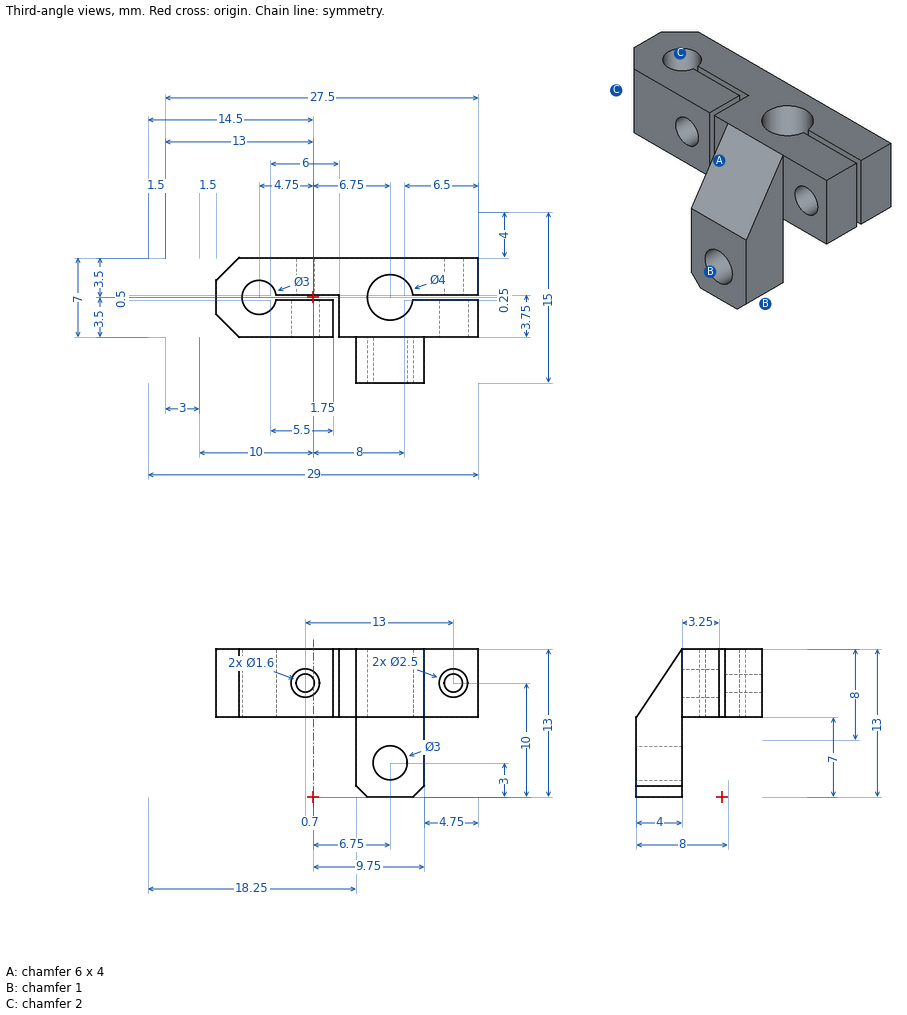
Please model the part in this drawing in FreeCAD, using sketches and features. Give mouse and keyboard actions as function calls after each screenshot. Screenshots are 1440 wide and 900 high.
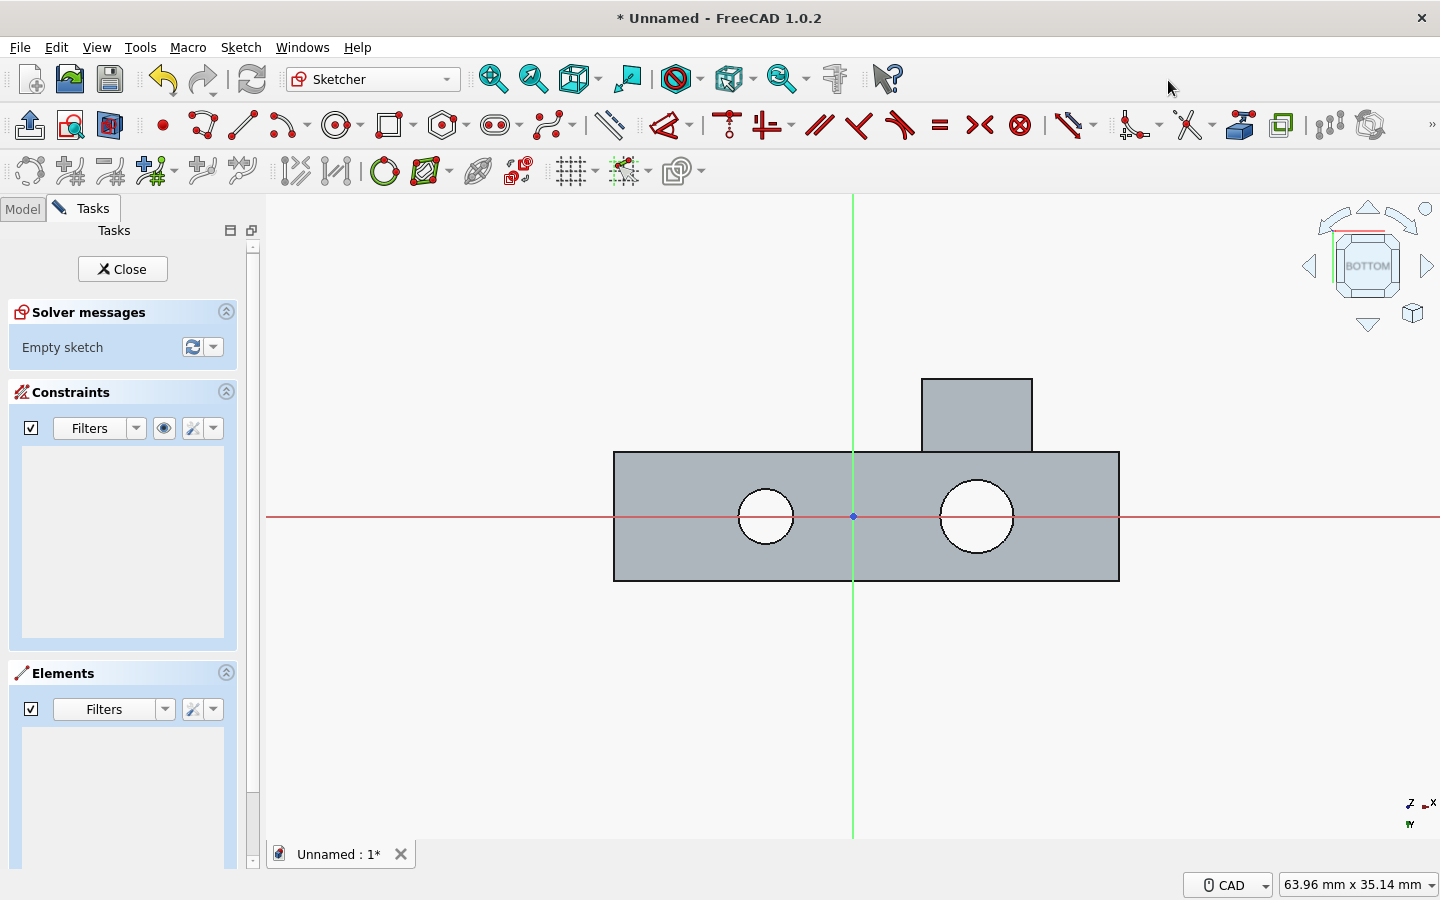
scroll(1088, 462, up, 4)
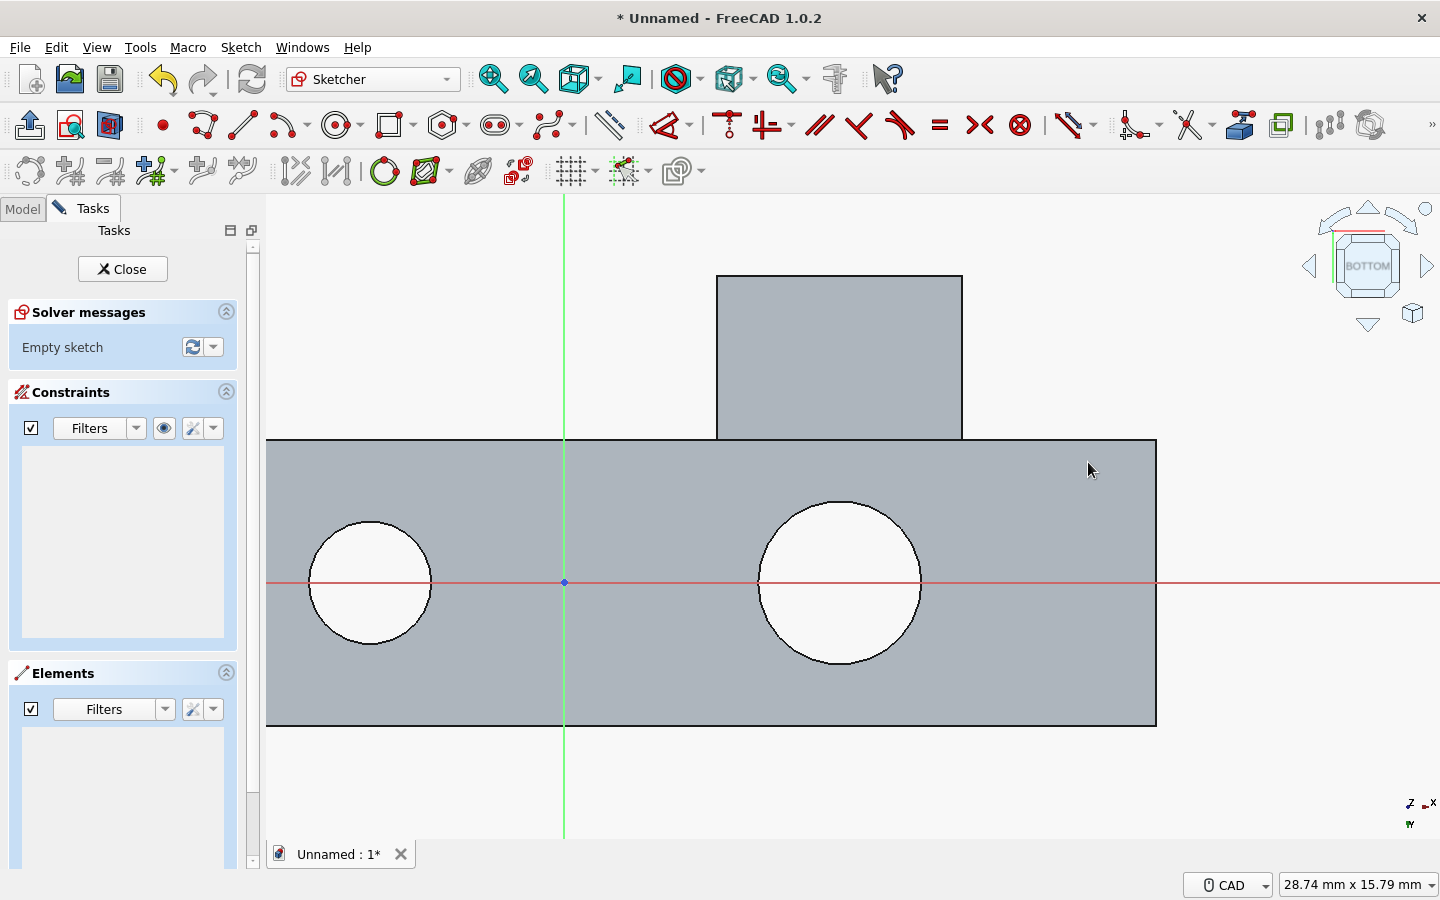
click(204, 126)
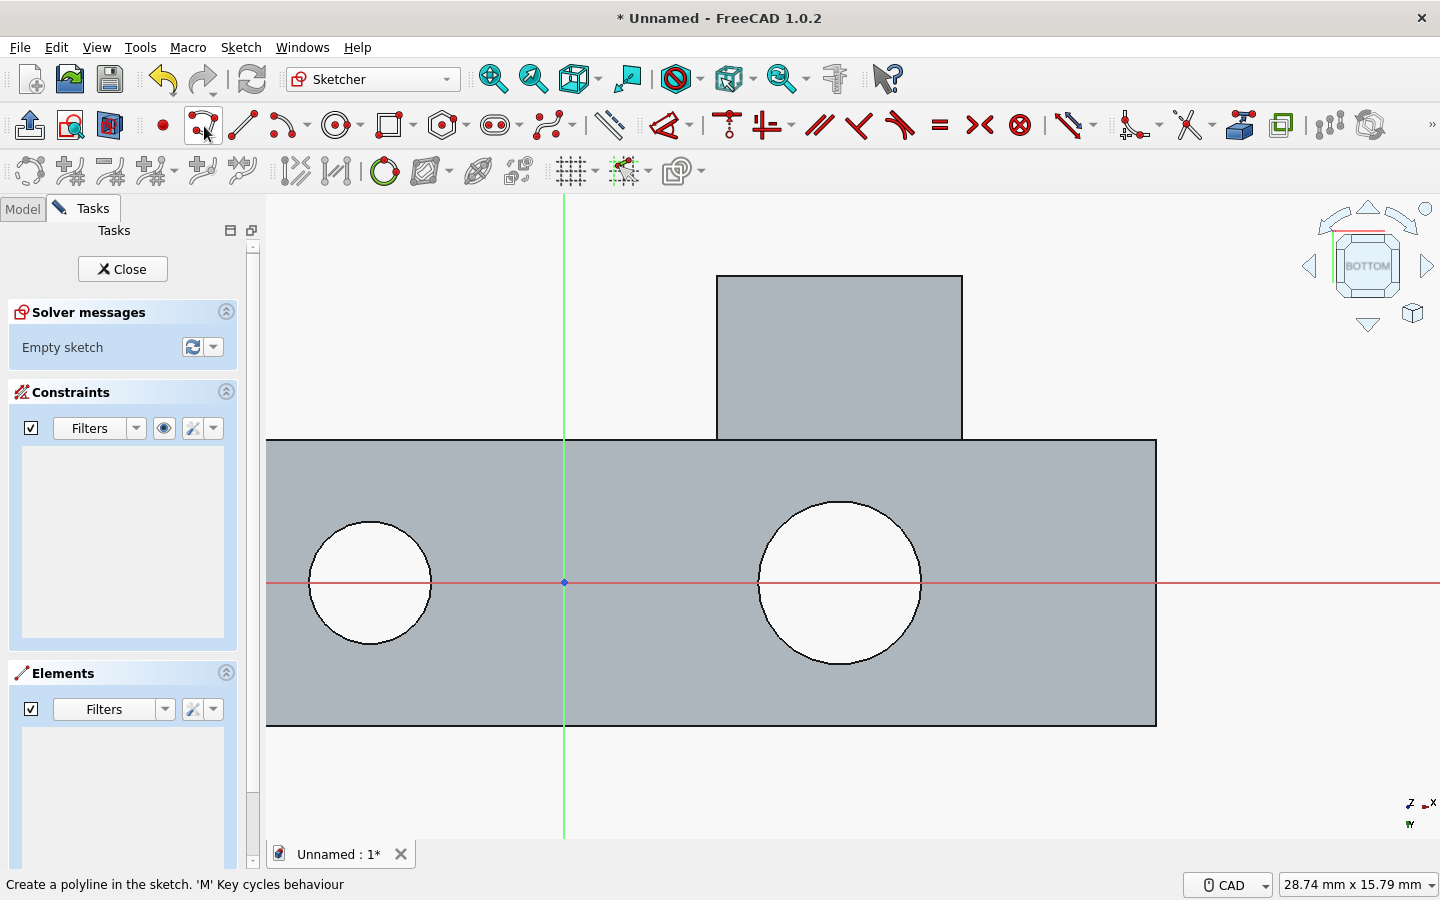
scroll(636, 573, up, 3)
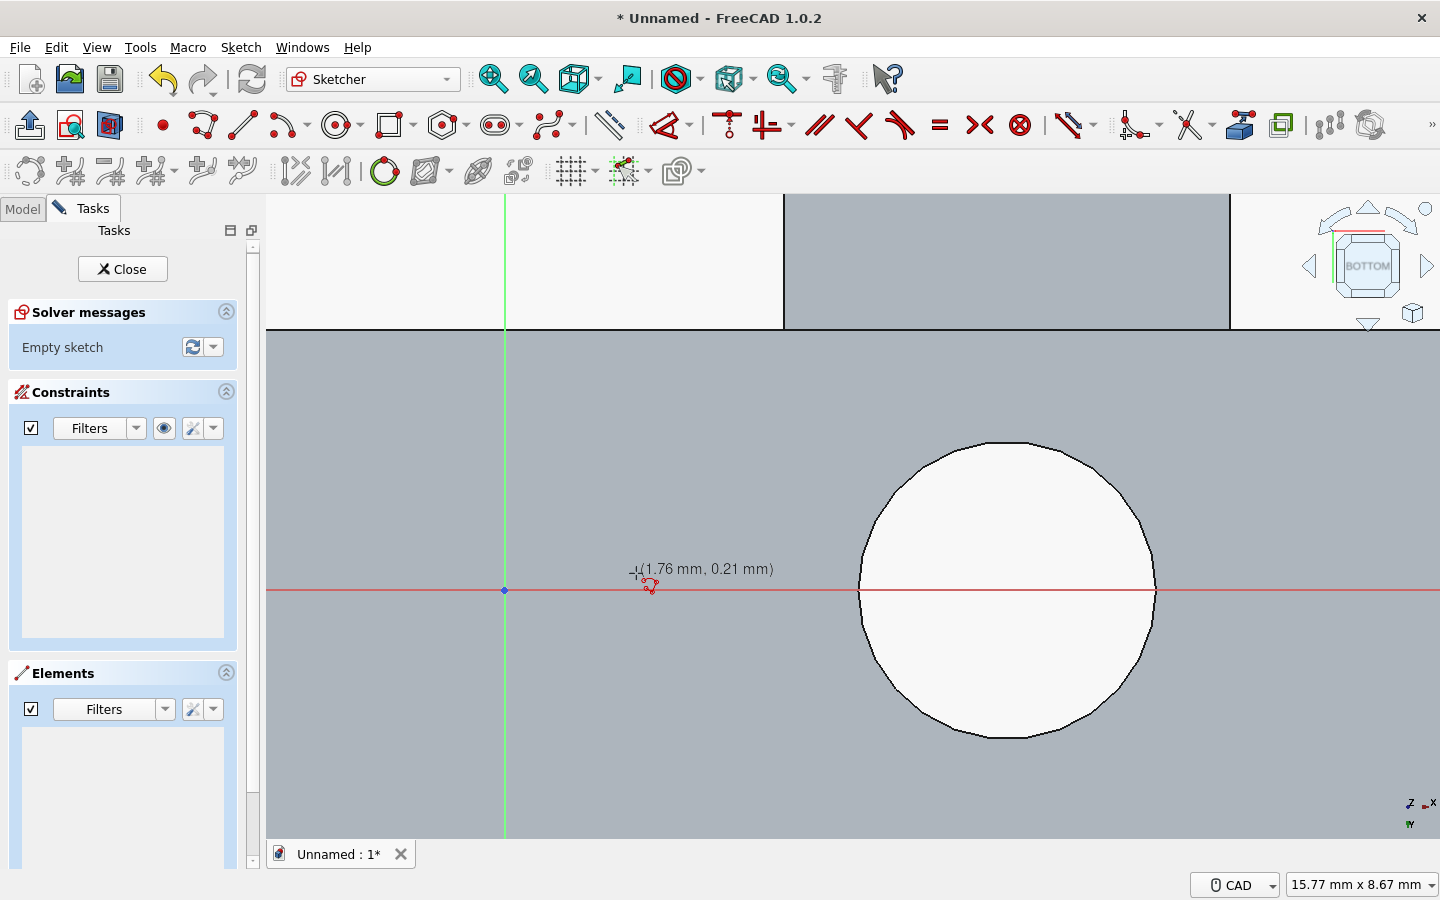
click(635, 572)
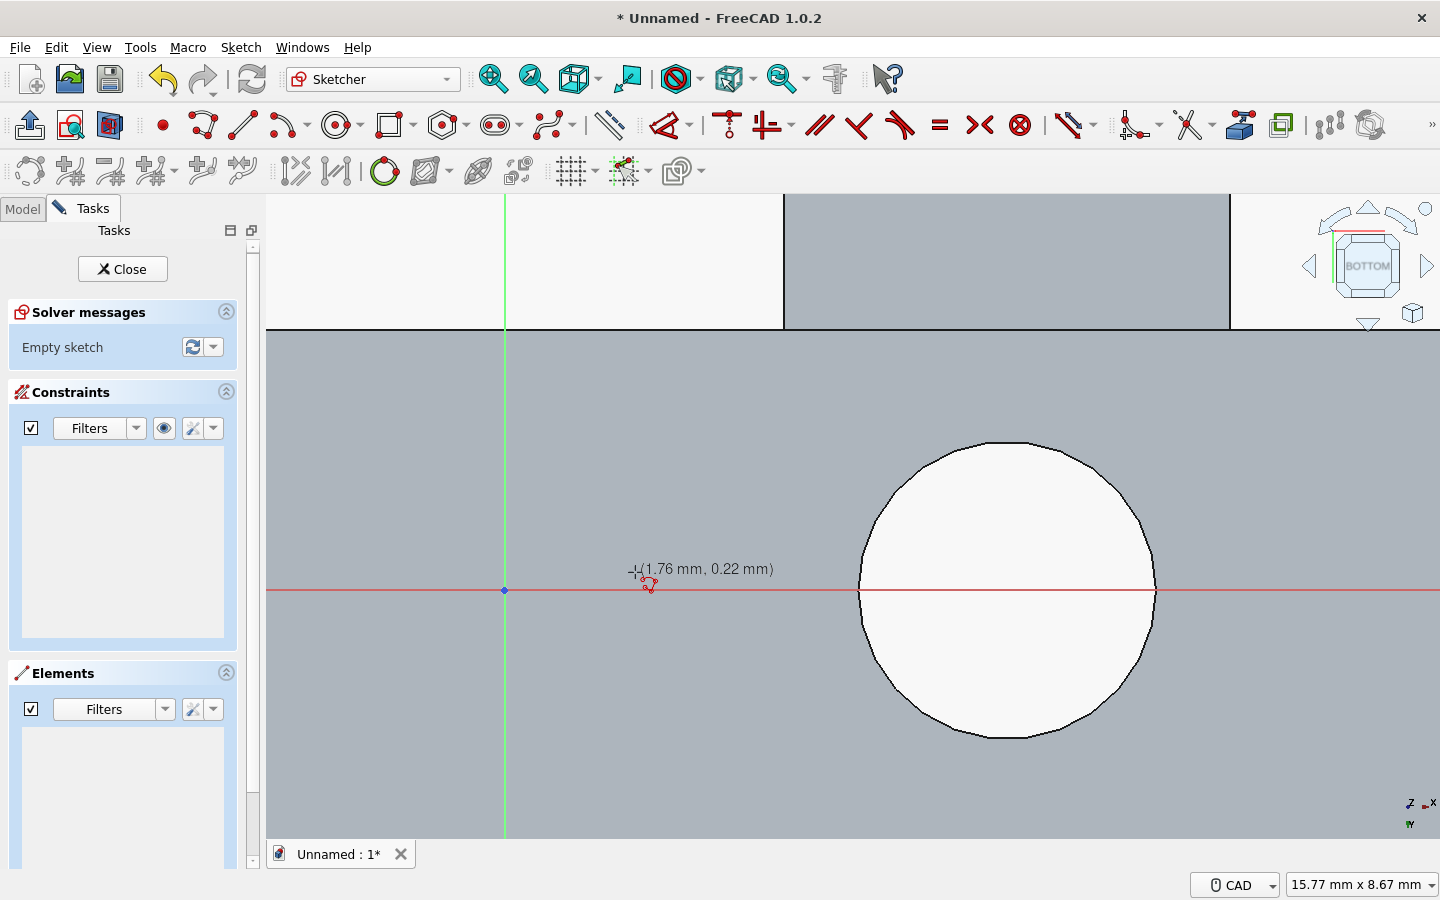
scroll(638, 574, down, 3)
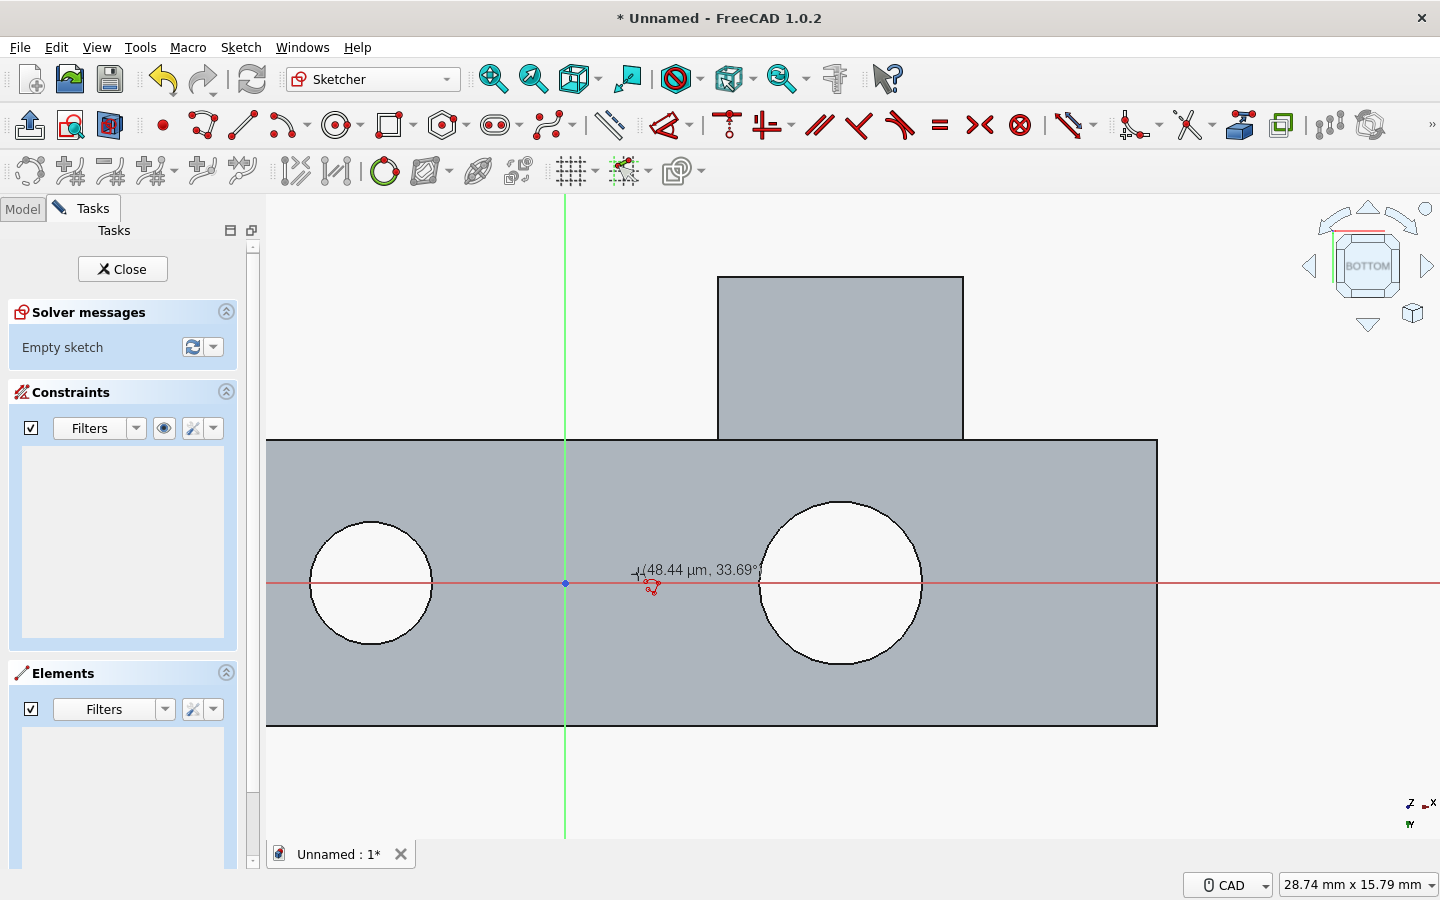
scroll(412, 573, up, 3)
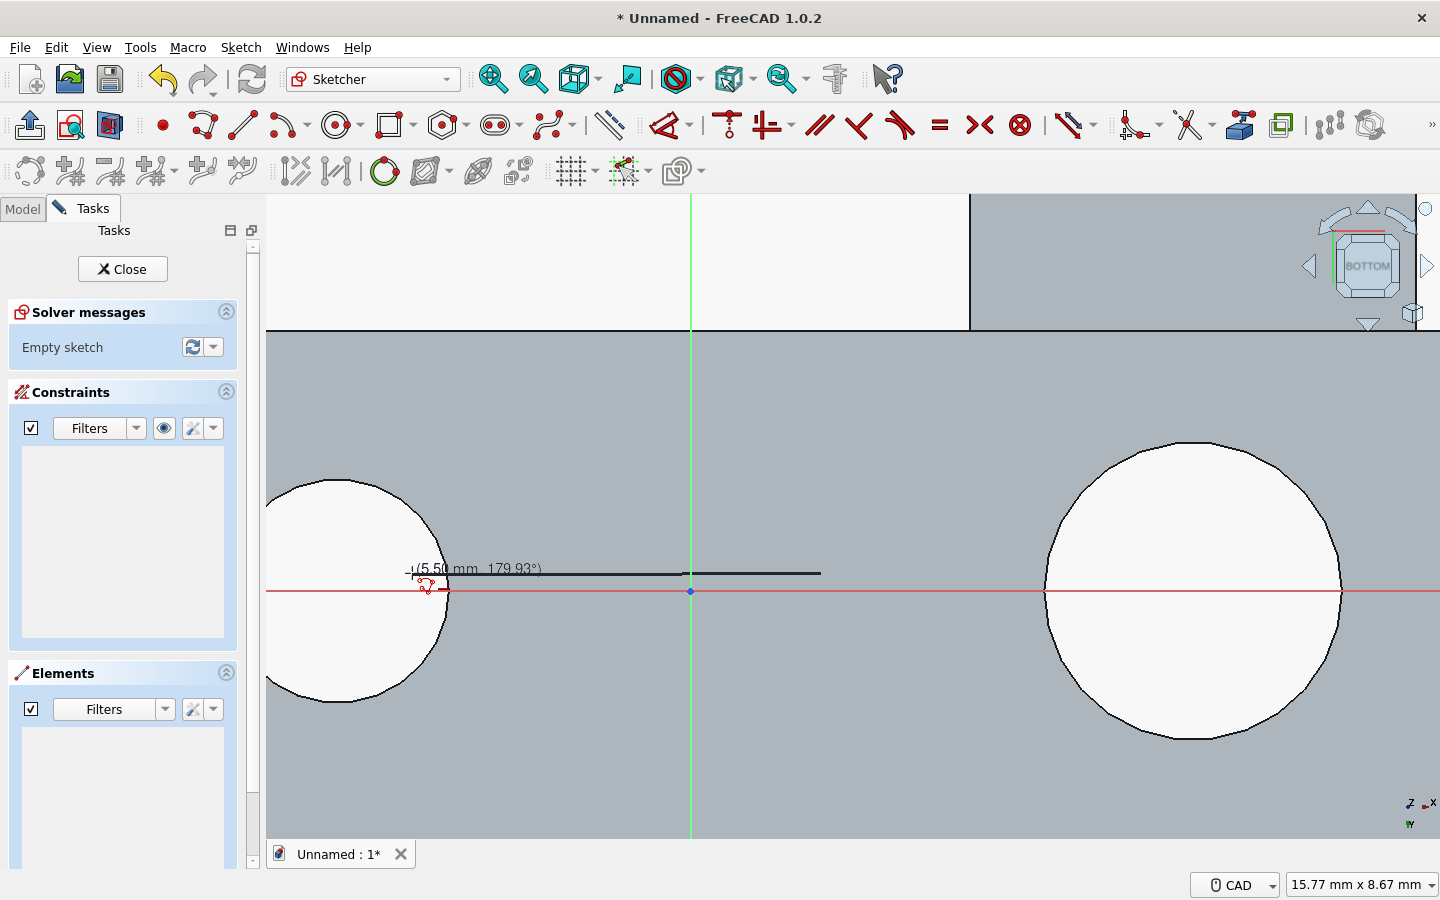
click(412, 573)
click(412, 610)
click(858, 610)
click(858, 331)
click(821, 331)
click(821, 574)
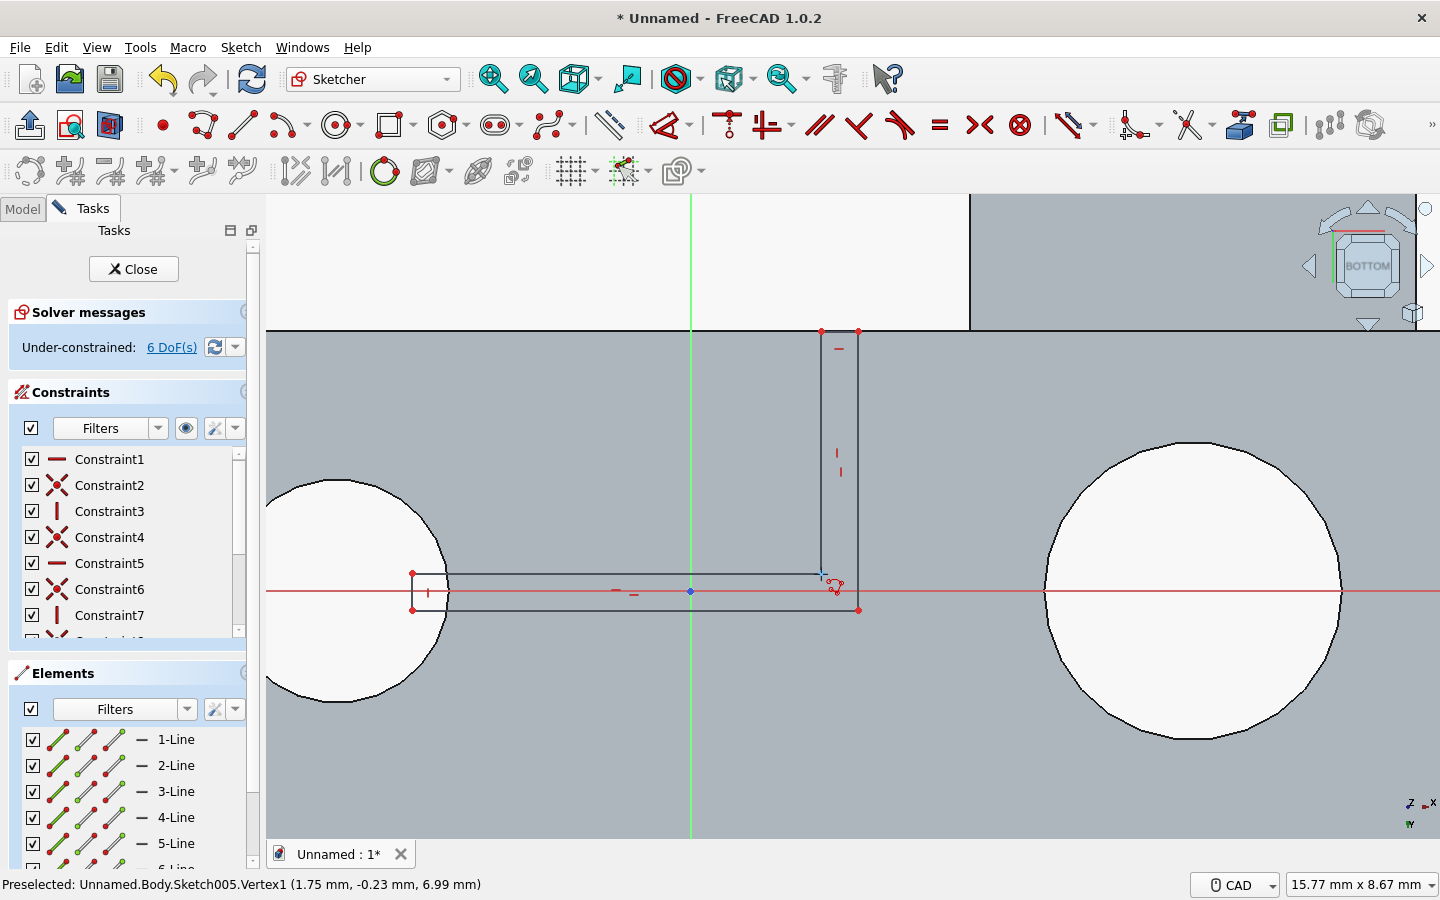
click(390, 126)